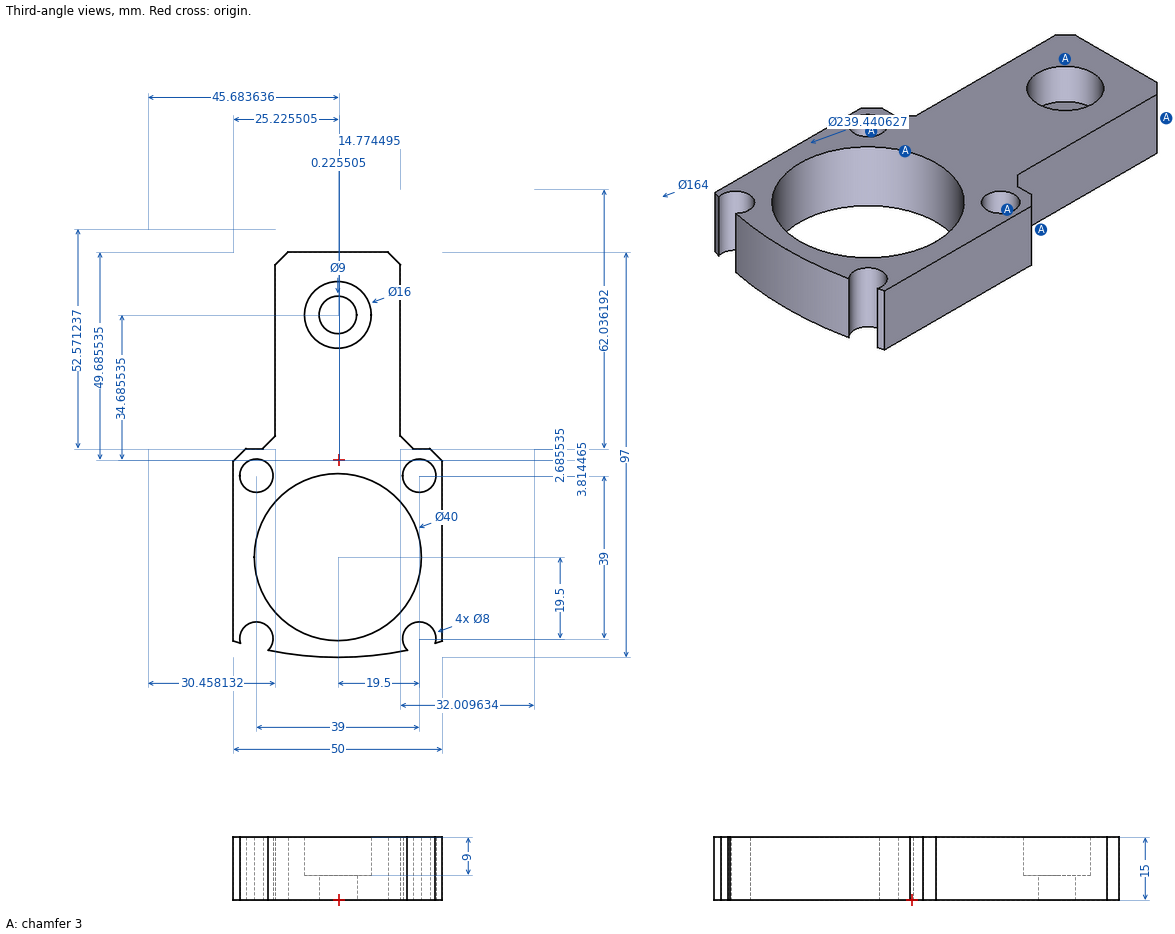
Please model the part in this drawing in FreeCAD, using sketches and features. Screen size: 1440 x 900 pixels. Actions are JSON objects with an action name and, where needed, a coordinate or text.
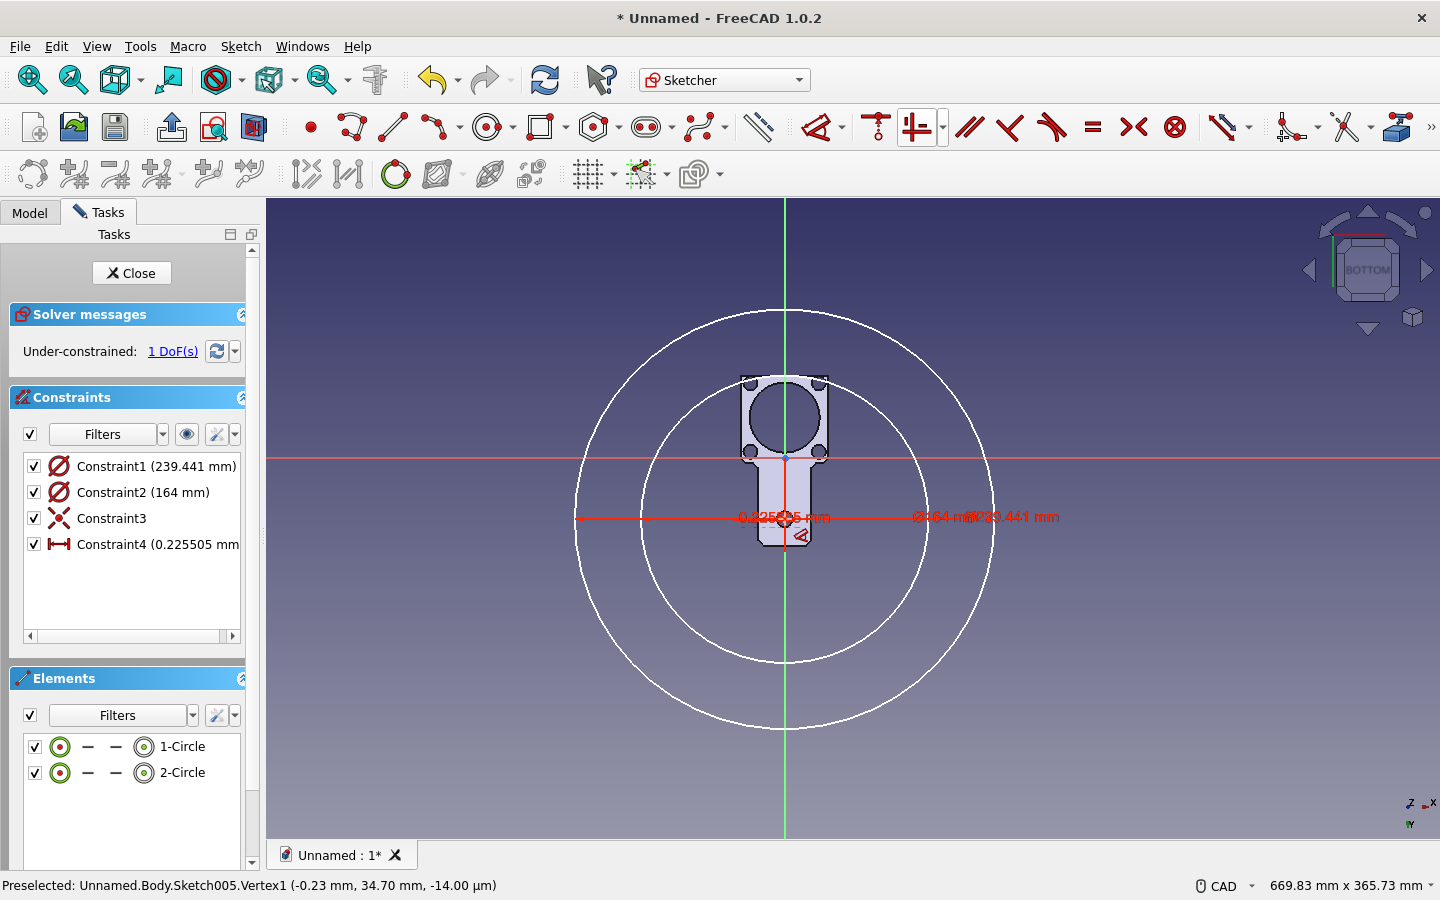
{"action": "left_click", "coordinate": [785, 519]}
{"action": "left_click", "coordinate": [819, 489]}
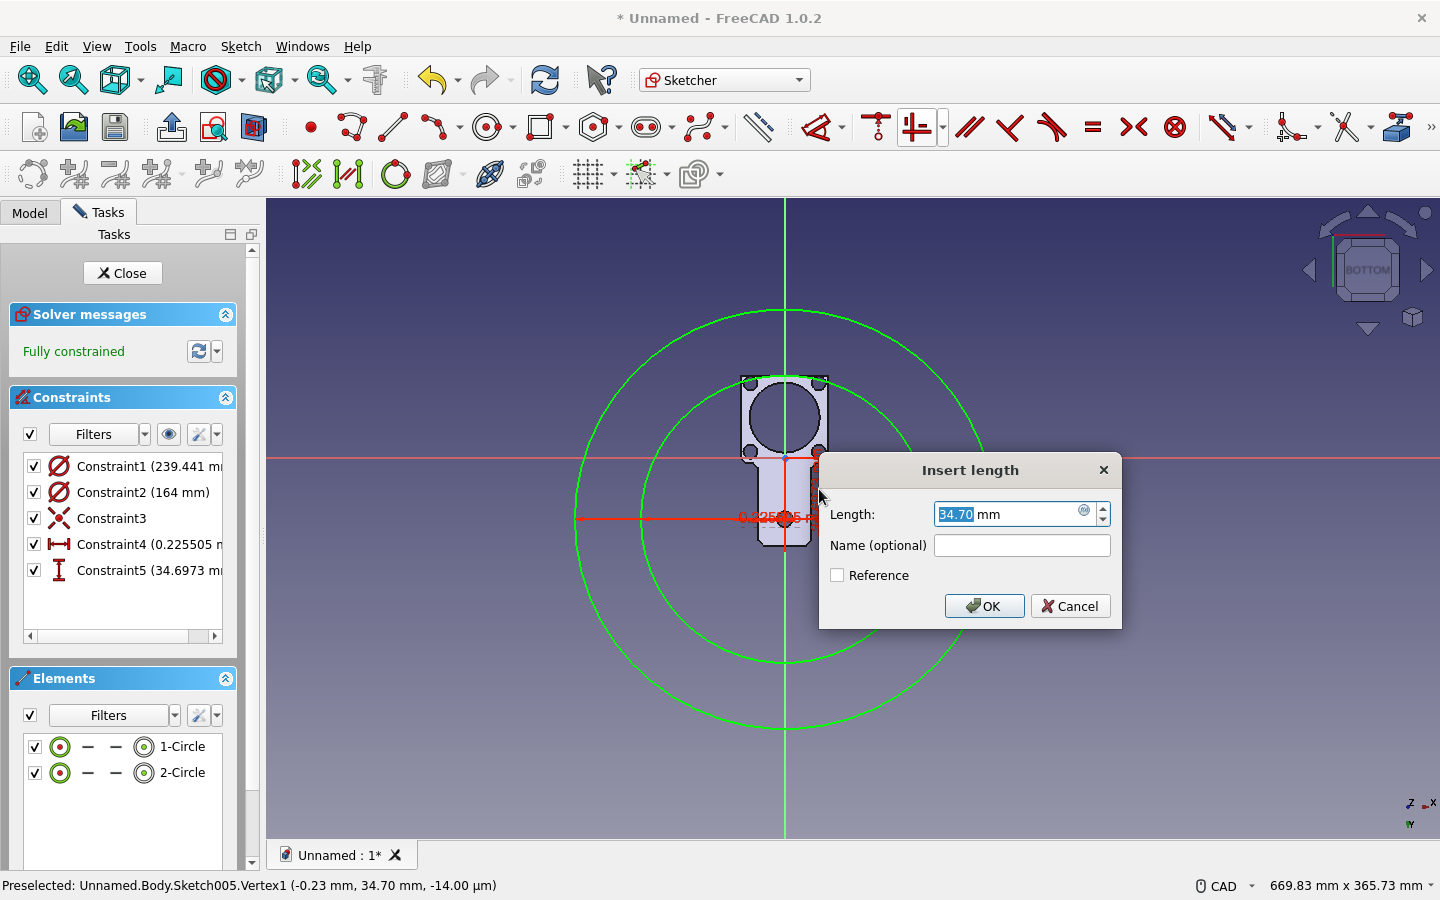
{"action": "type", "text": "34.685535"}
{"action": "key", "text": "Return"}
{"action": "key", "text": "Escape"}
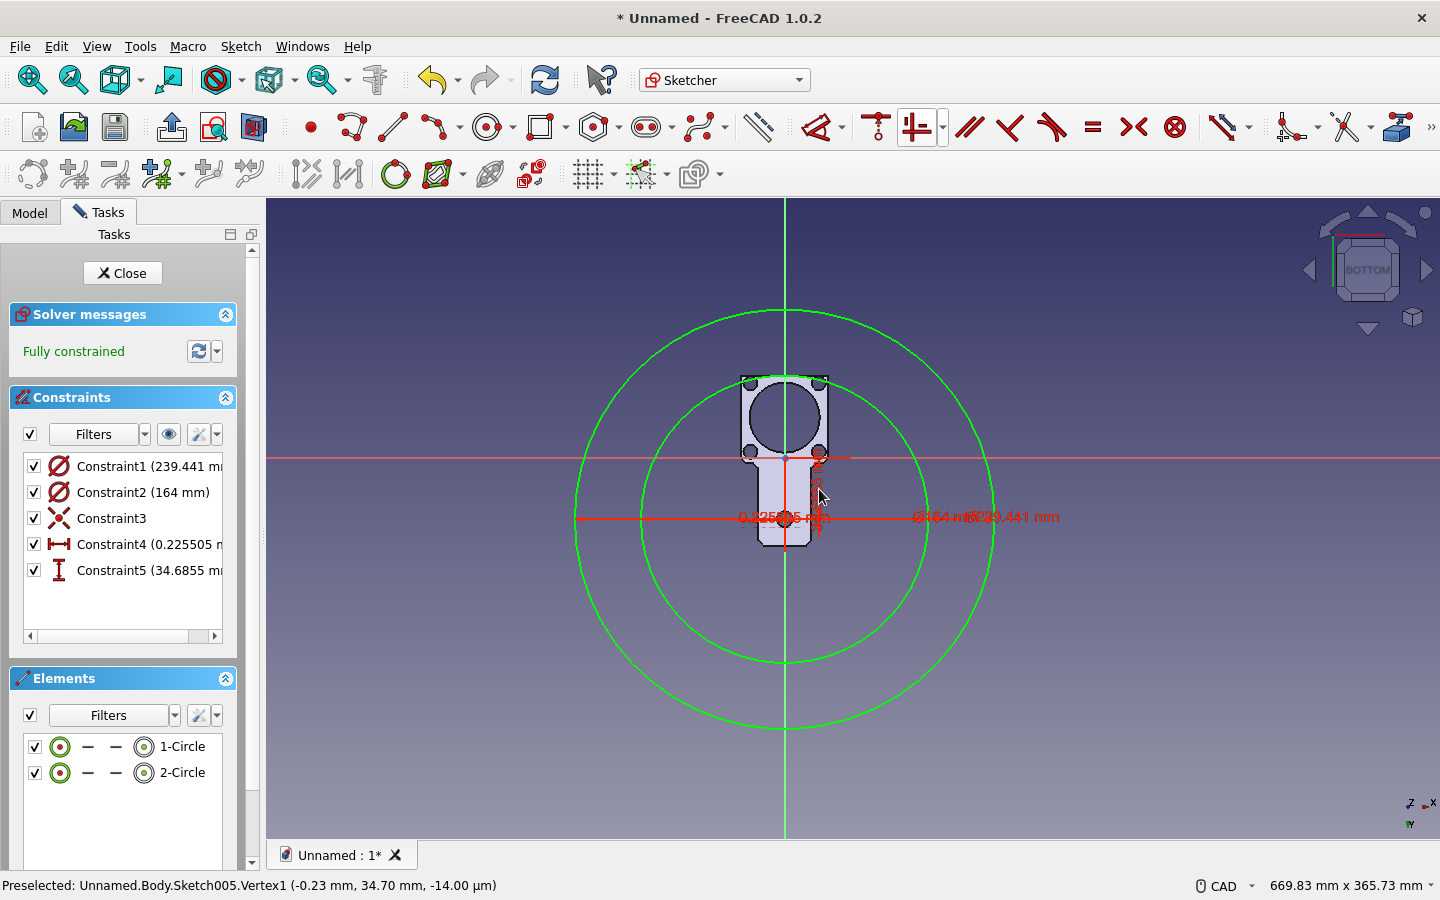
{"action": "left_click", "coordinate": [123, 273]}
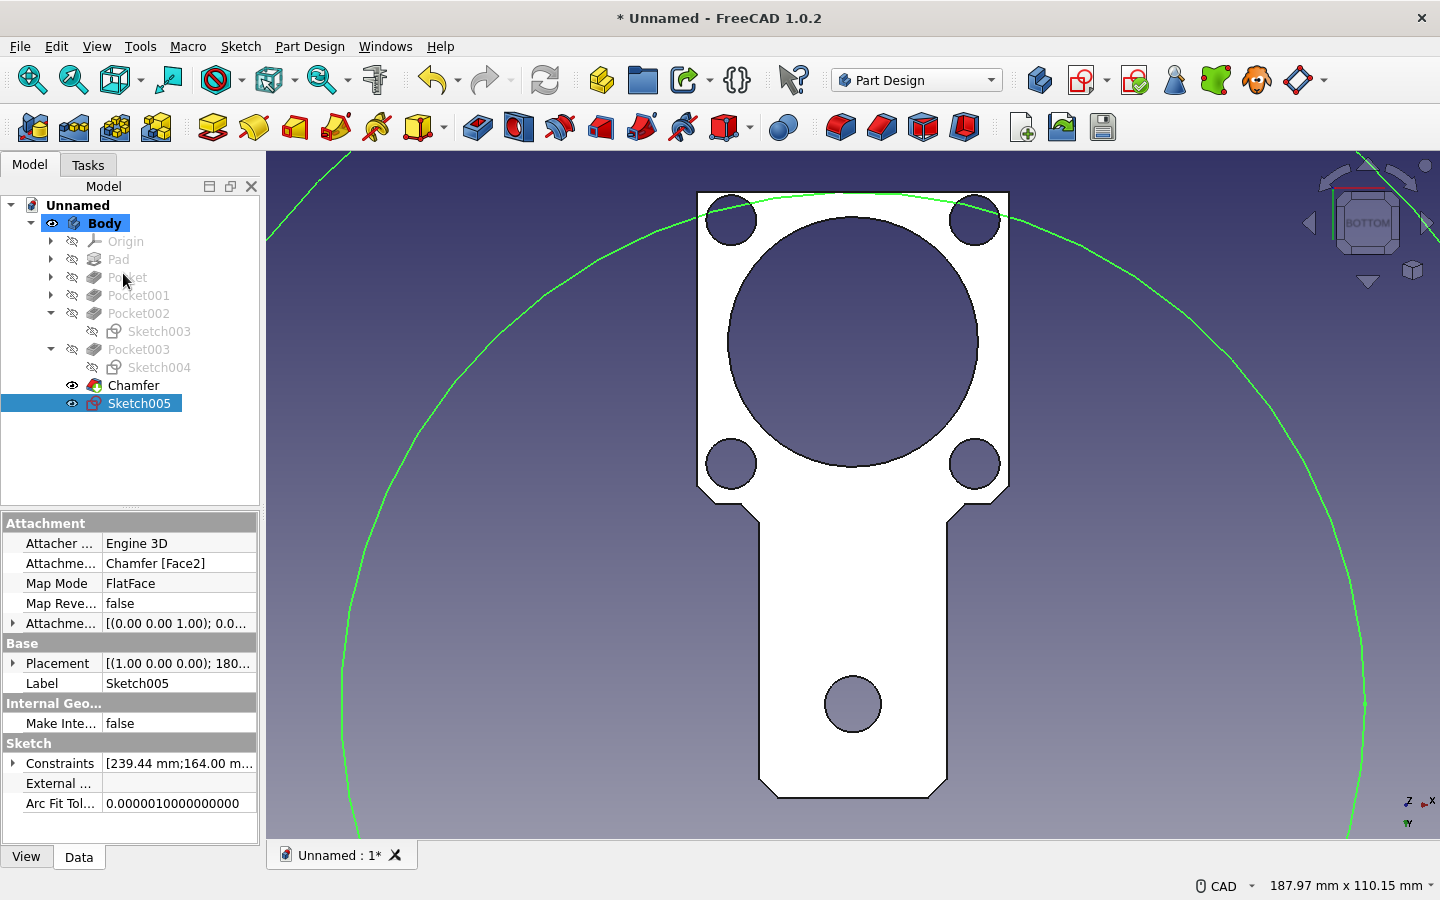
{"action": "left_click", "coordinate": [478, 128]}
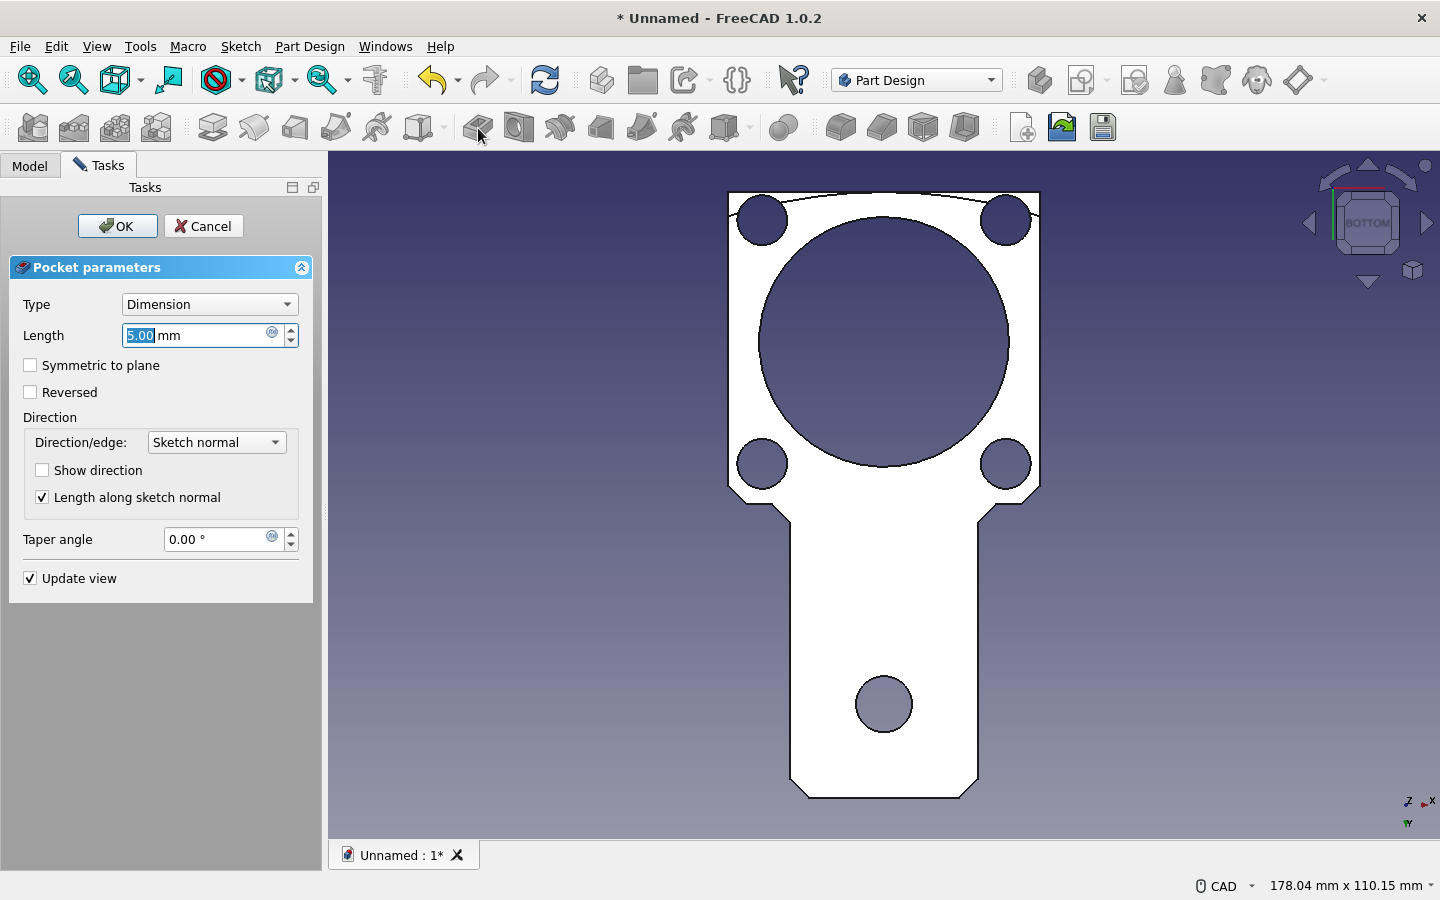
{"action": "left_click", "coordinate": [210, 304]}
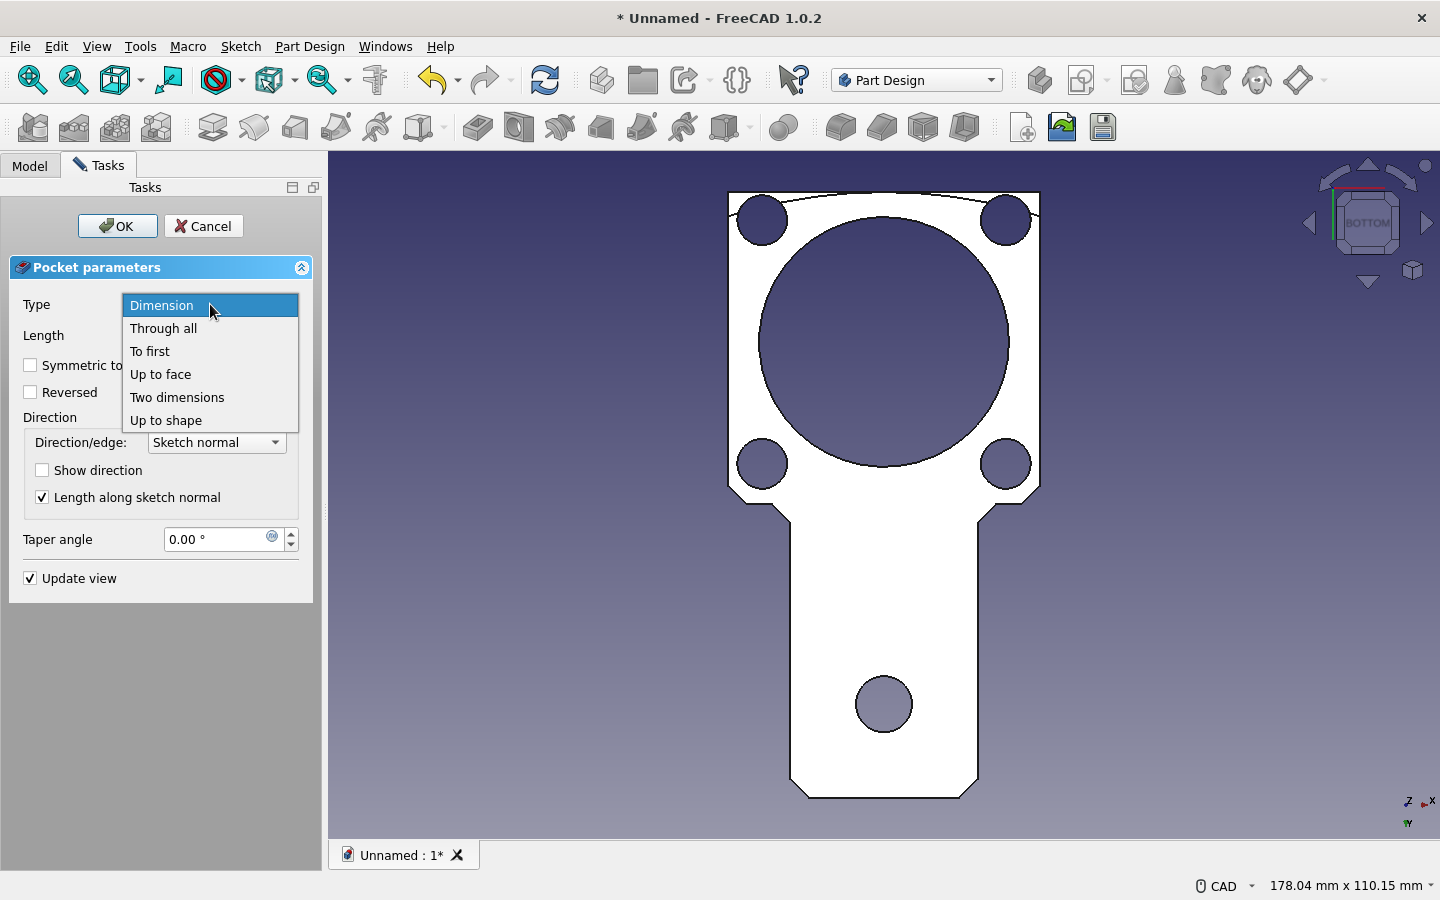
{"action": "left_click", "coordinate": [208, 328]}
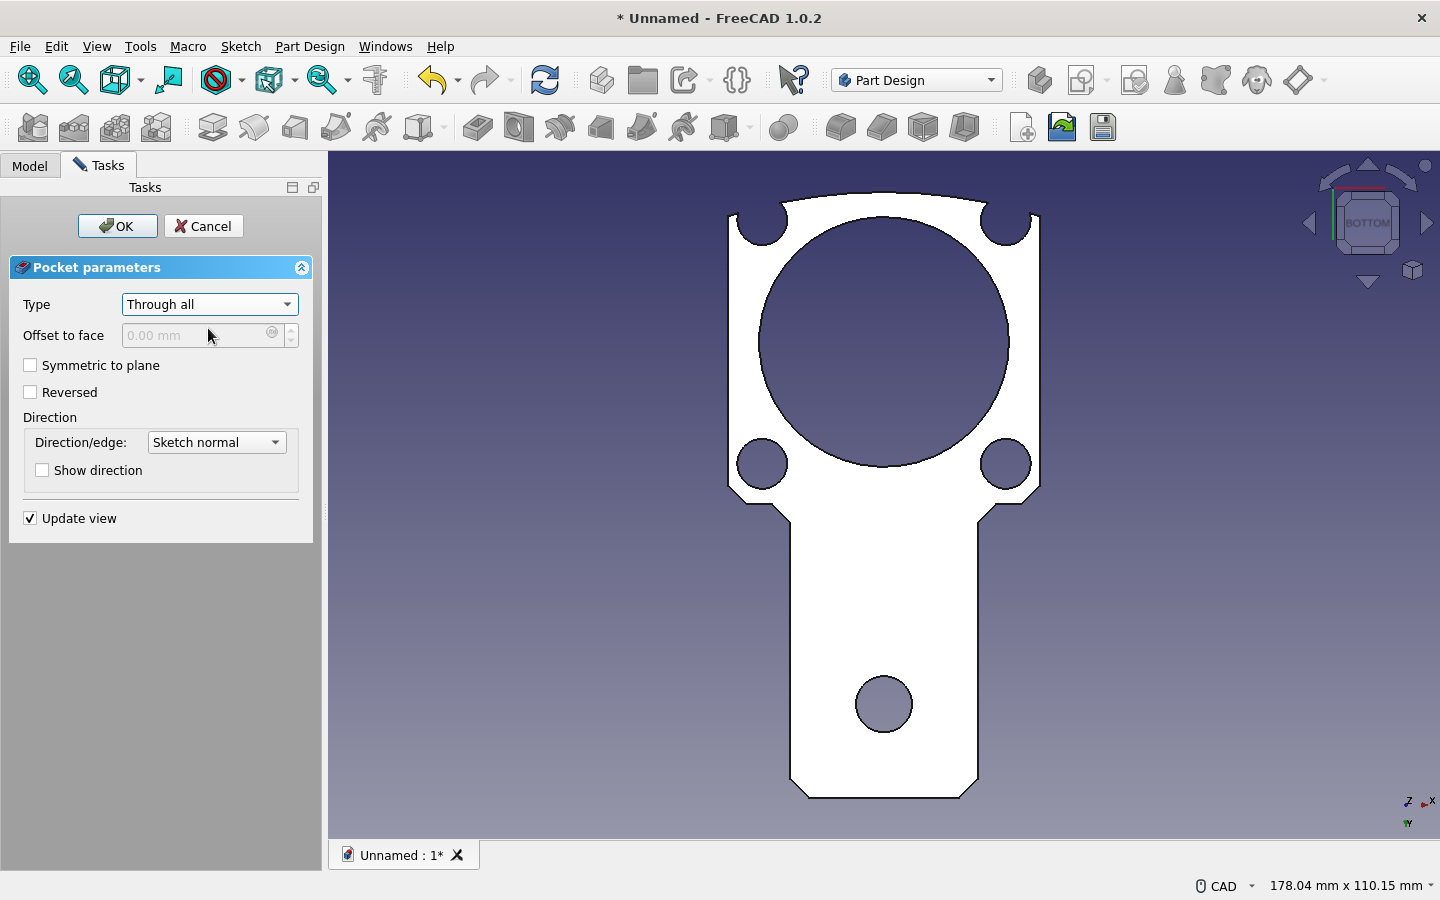
{"action": "left_click", "coordinate": [118, 226]}